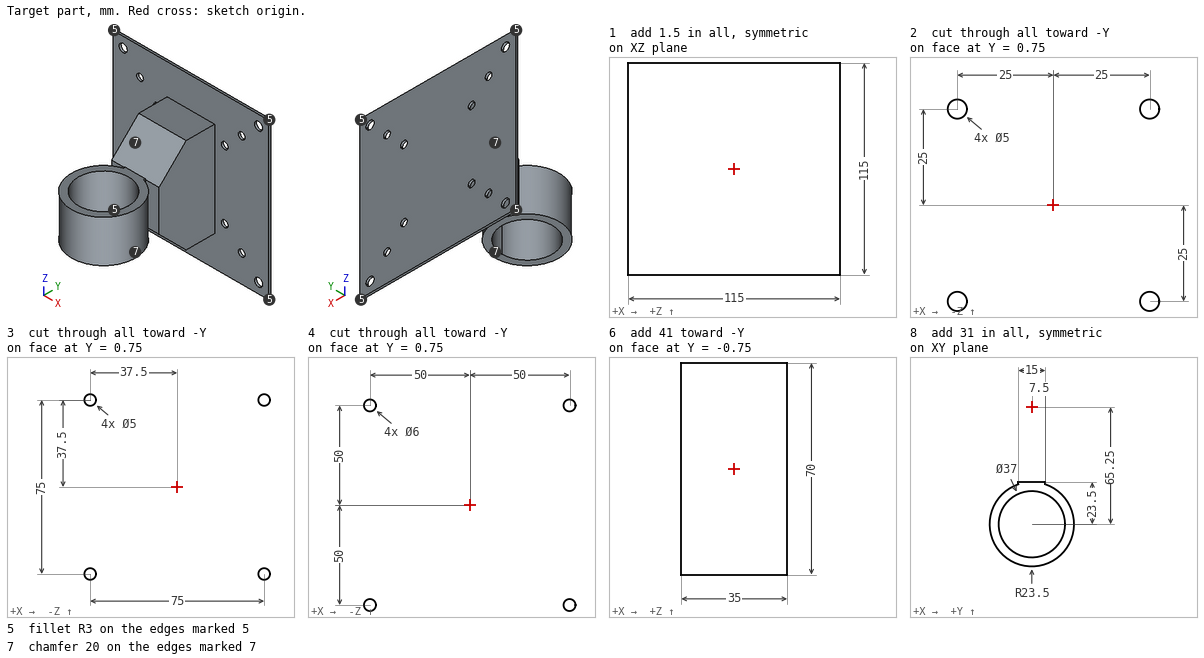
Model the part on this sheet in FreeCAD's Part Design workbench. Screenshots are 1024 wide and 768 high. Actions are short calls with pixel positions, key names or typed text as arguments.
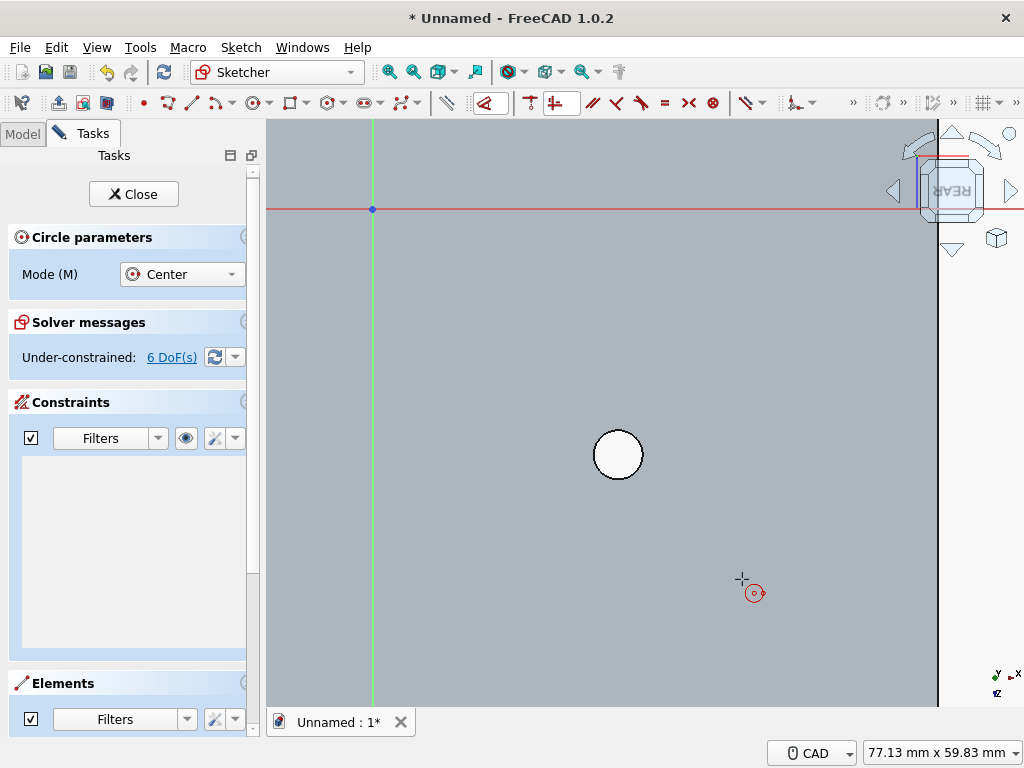
click(741, 578)
click(758, 560)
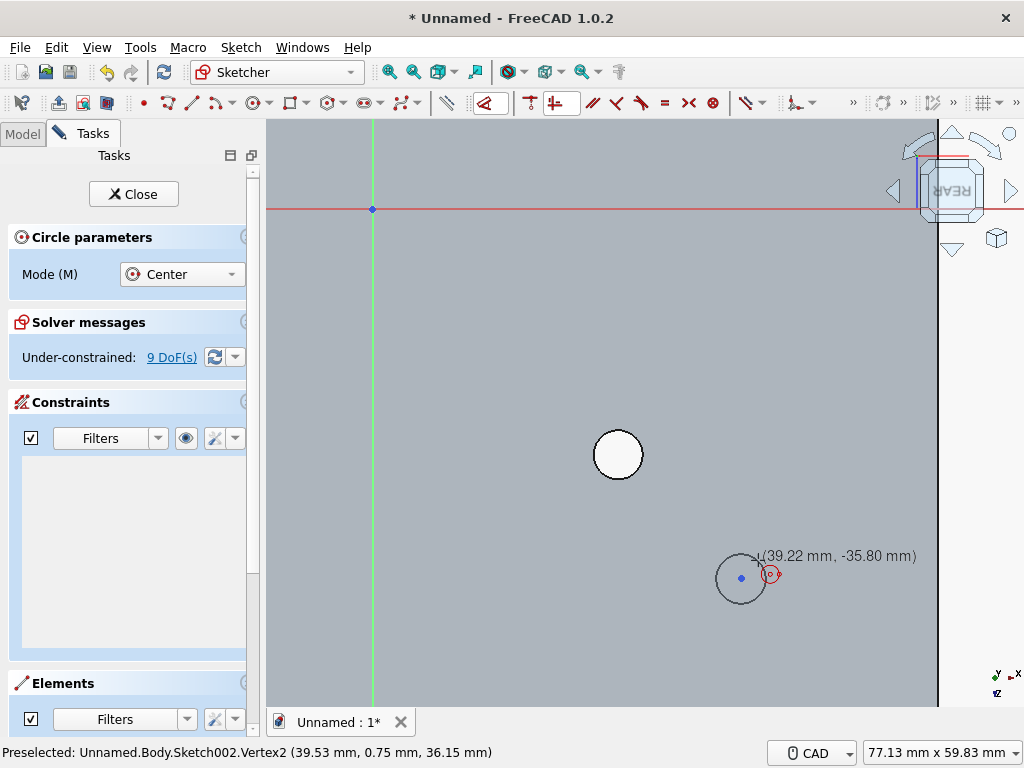
scroll(743, 579, down, 4)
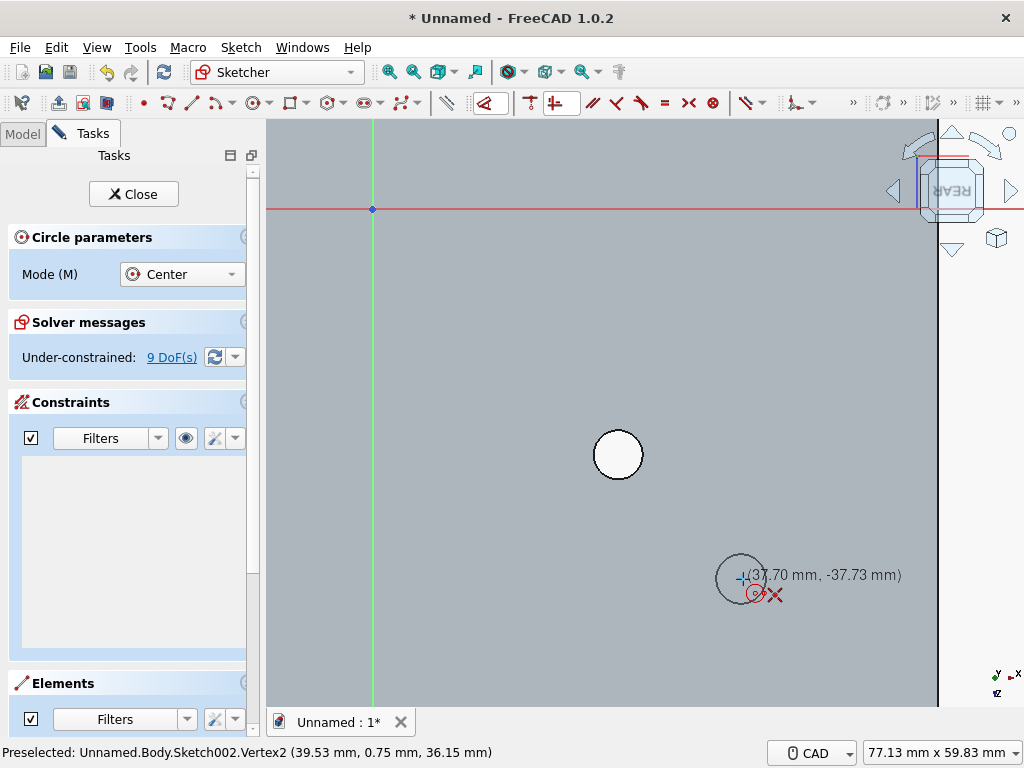
scroll(742, 248, up, 4)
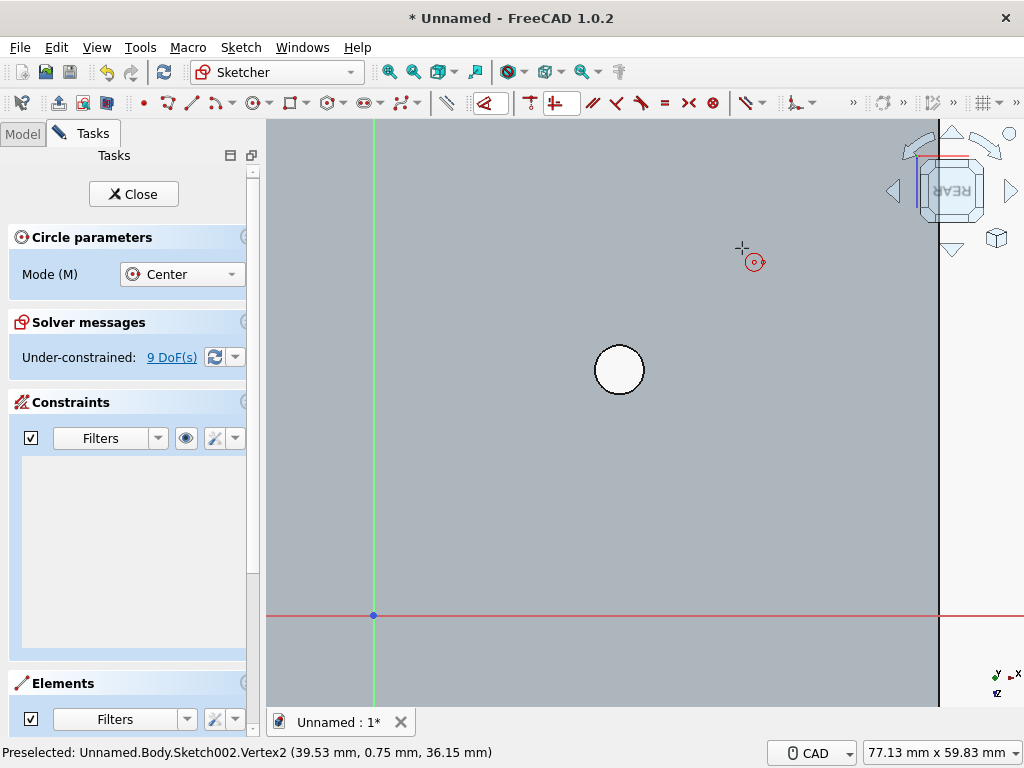
click(742, 247)
click(760, 230)
key(Escape)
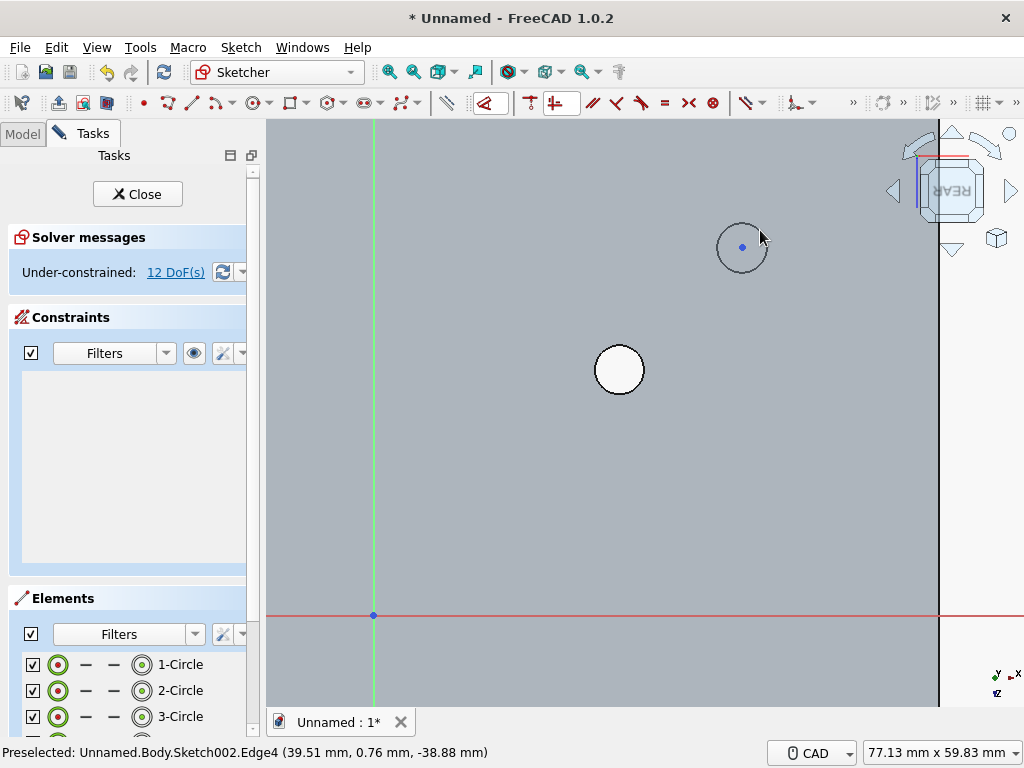
scroll(742, 248, down, 4)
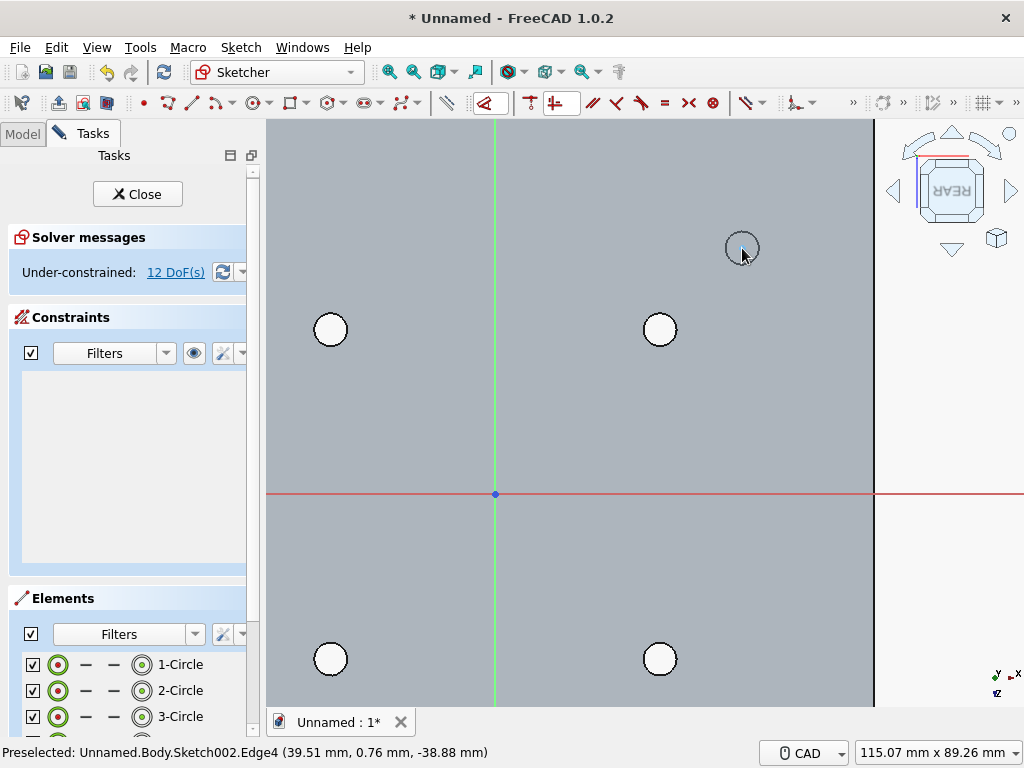
scroll(419, 240, up, 2)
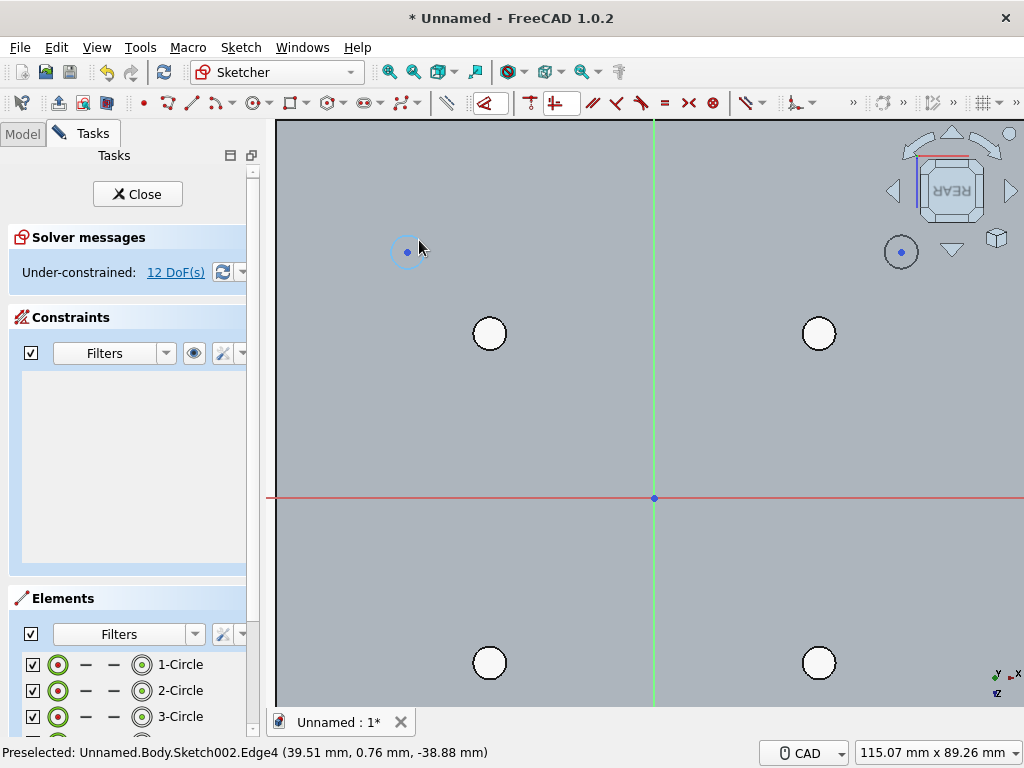
click(419, 240)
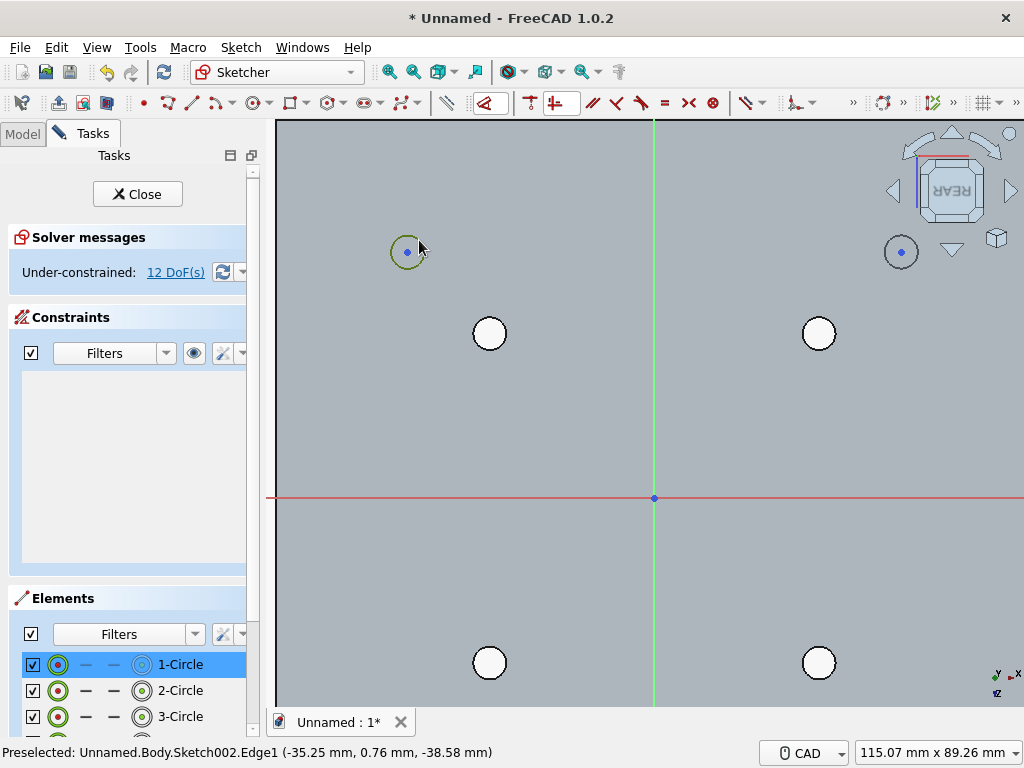
scroll(418, 239, down, 2)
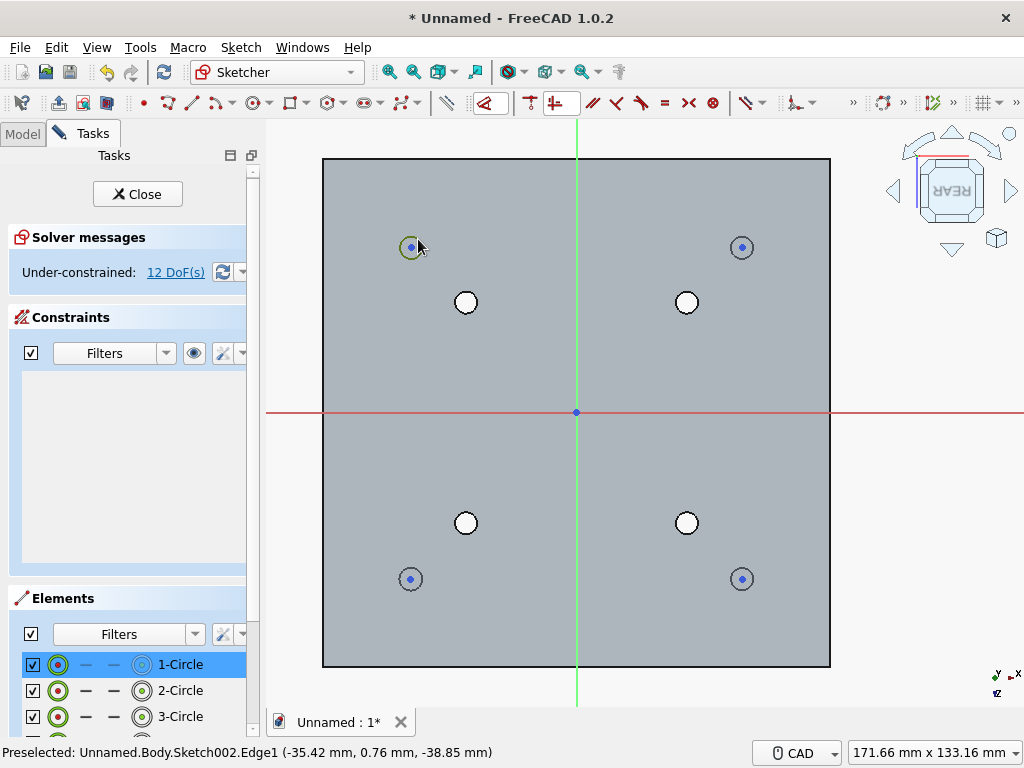
click(419, 571)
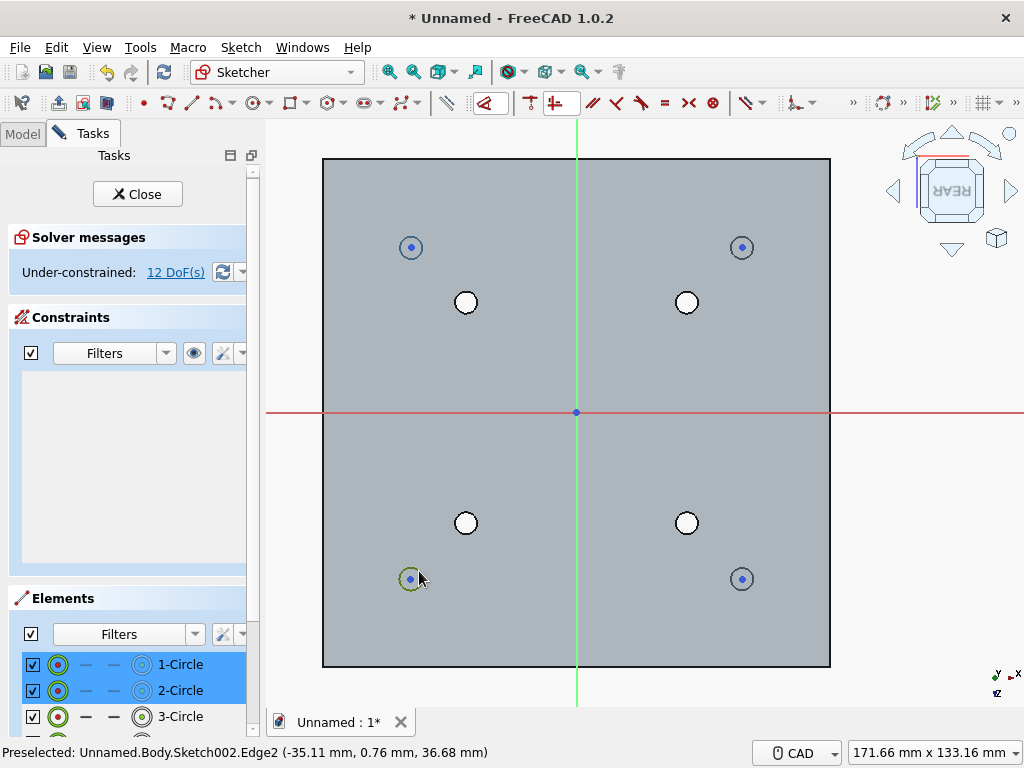
scroll(750, 571, up, 2)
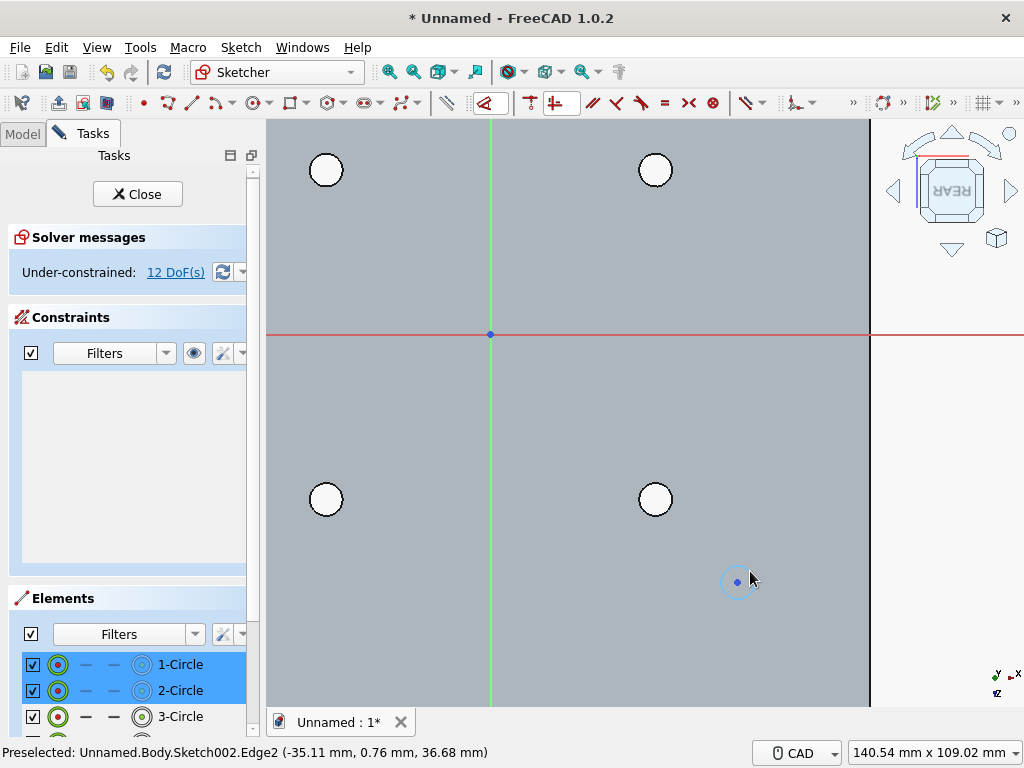
click(750, 571)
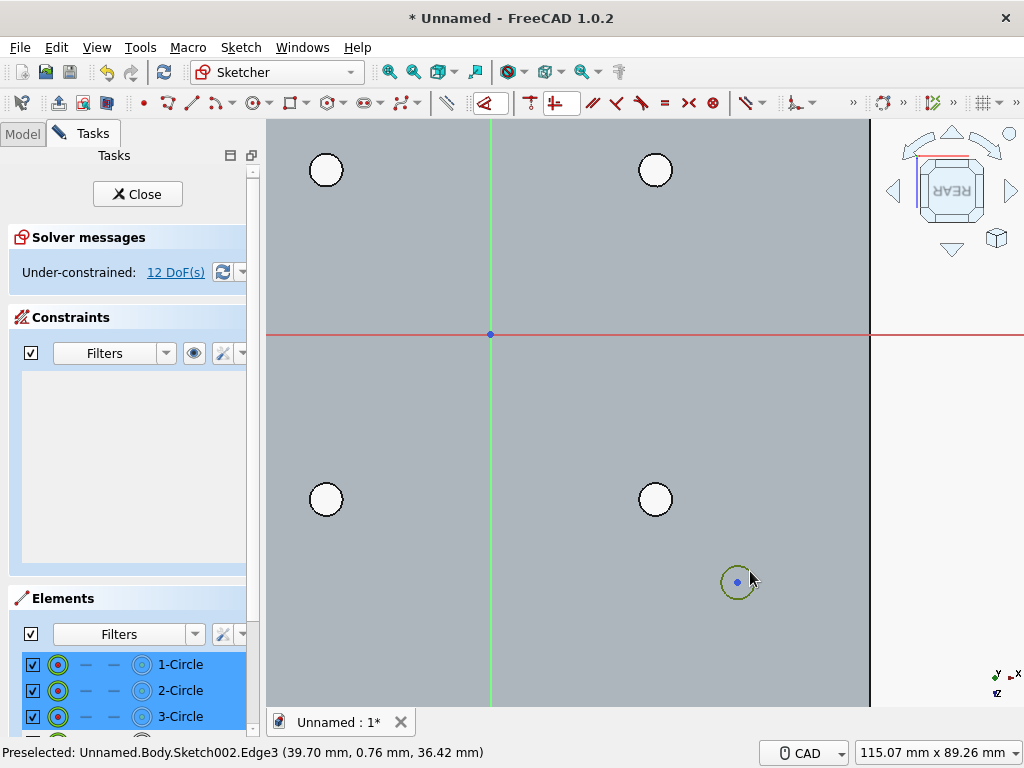
scroll(750, 572, down, 2)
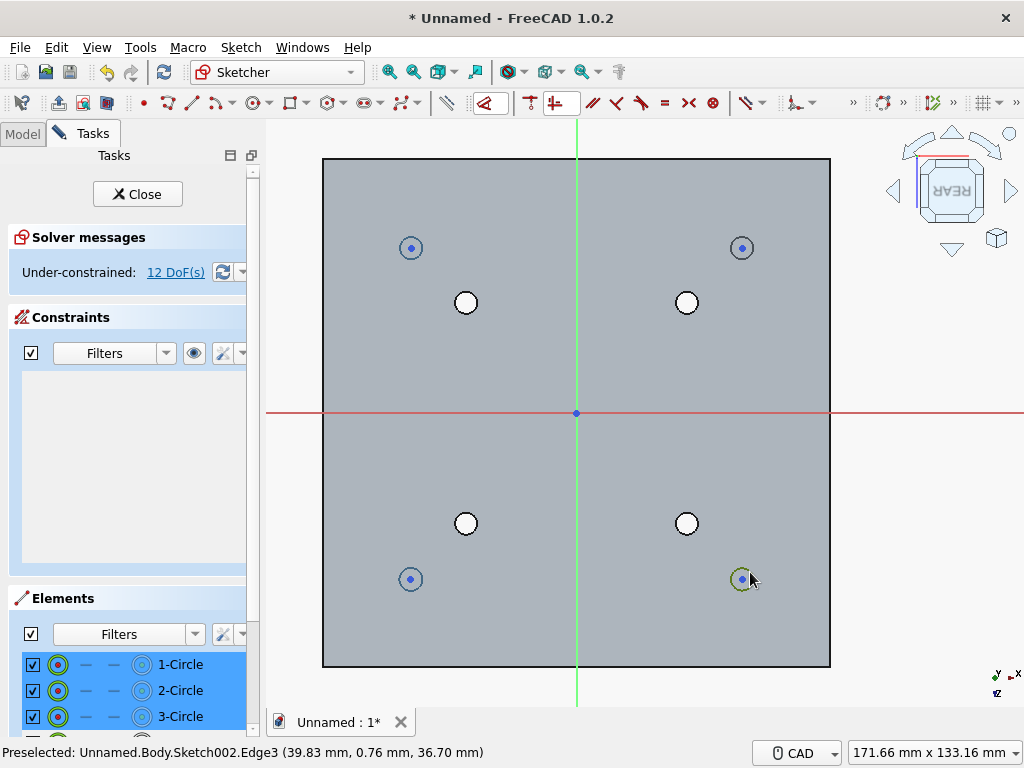
scroll(750, 240, up, 2)